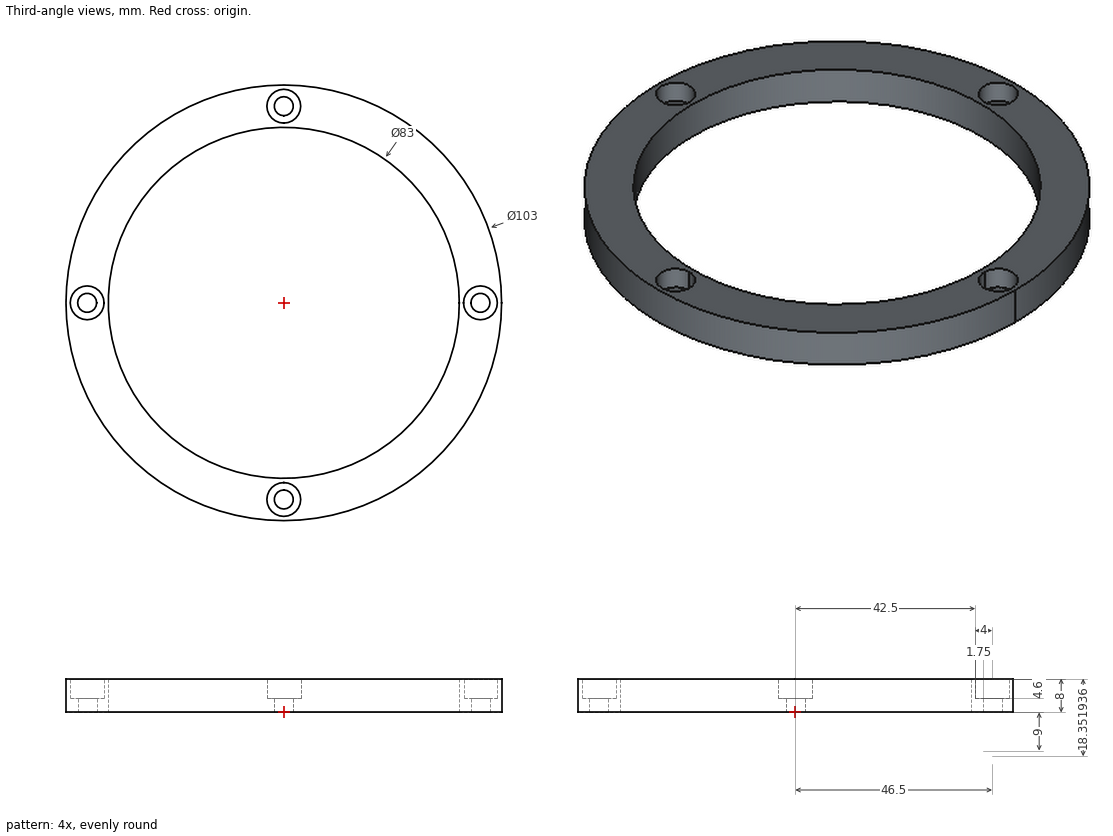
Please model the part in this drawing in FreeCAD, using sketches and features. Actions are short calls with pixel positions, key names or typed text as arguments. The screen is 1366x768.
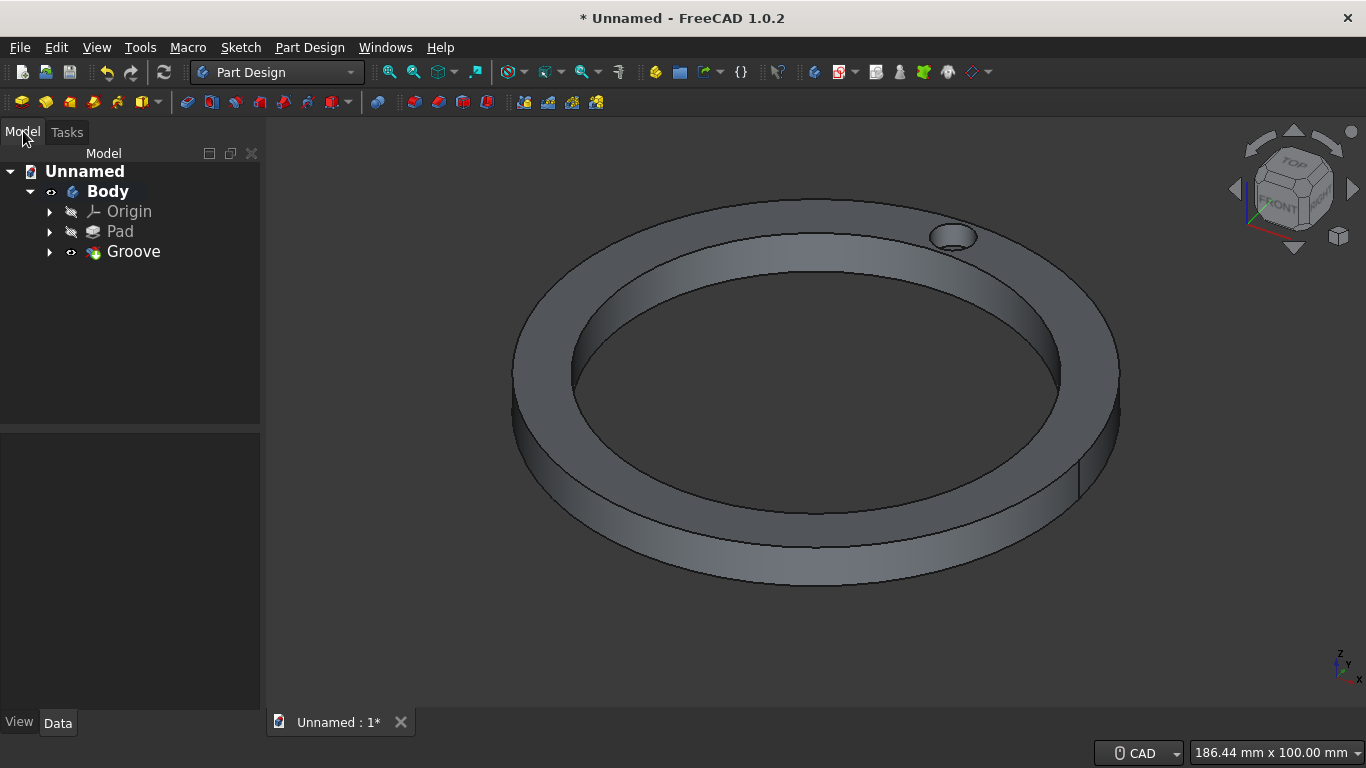
click(116, 252)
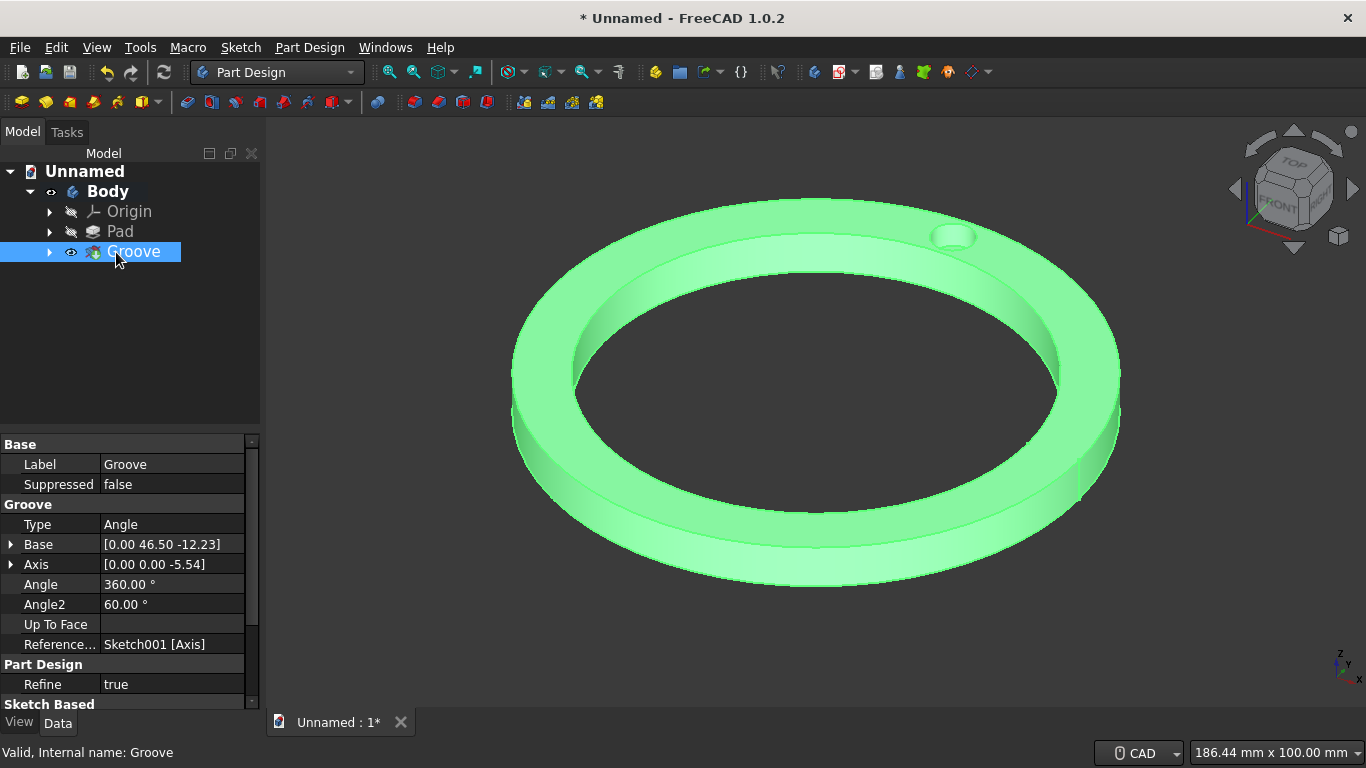
click(572, 102)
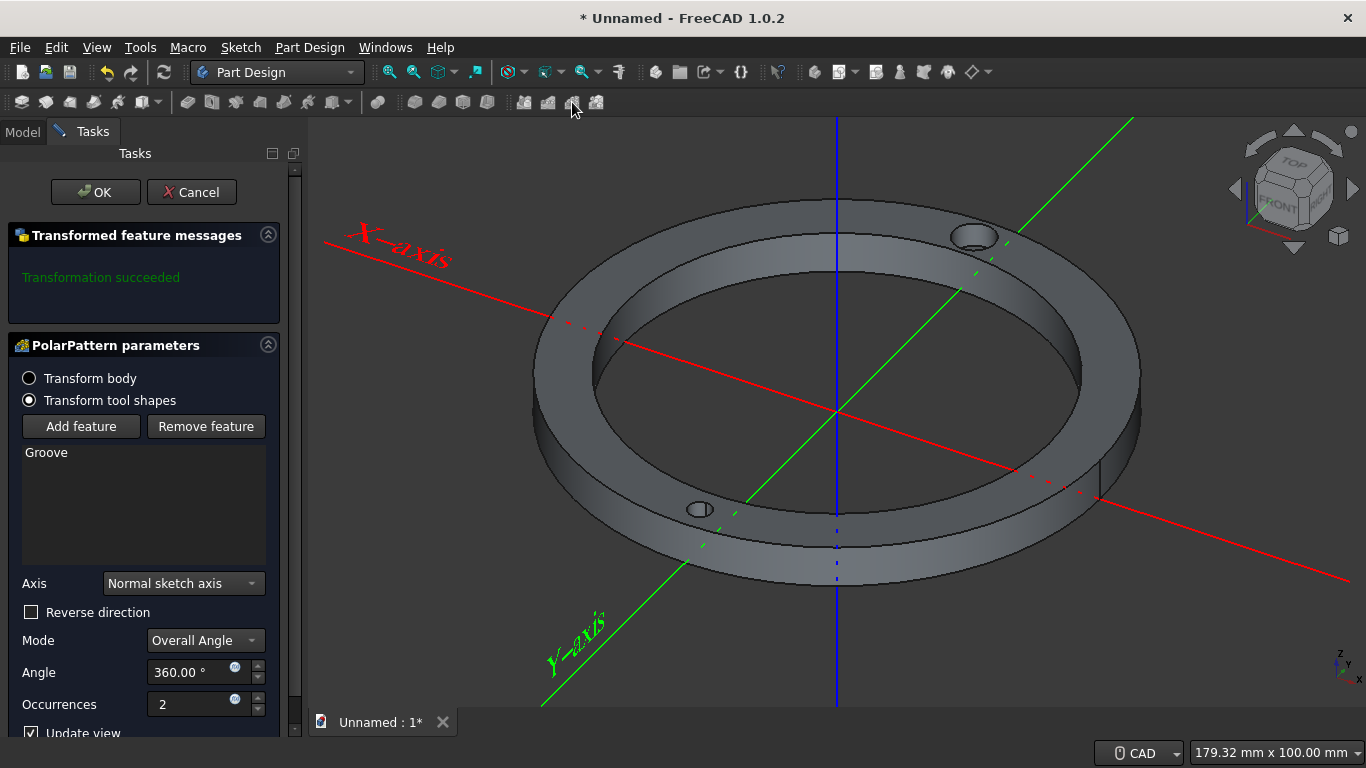
click(184, 584)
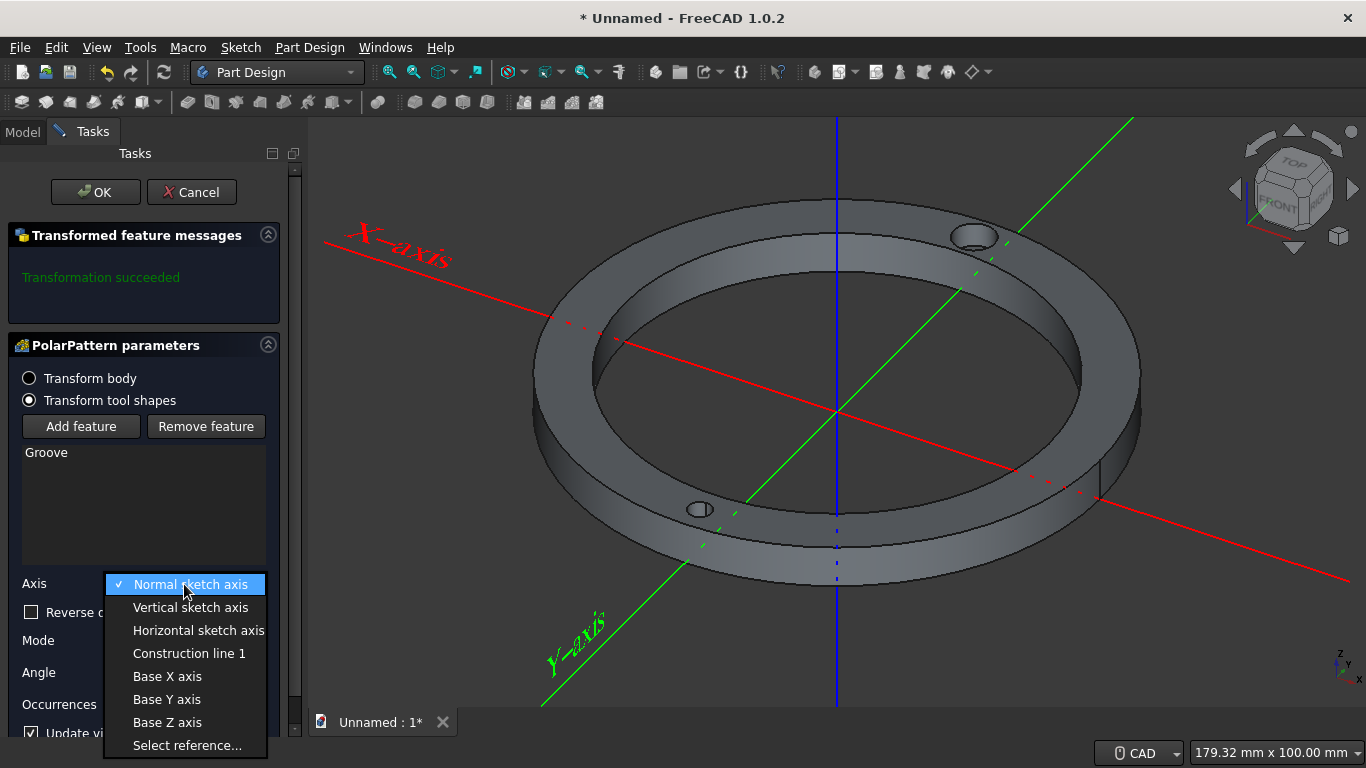
click(184, 722)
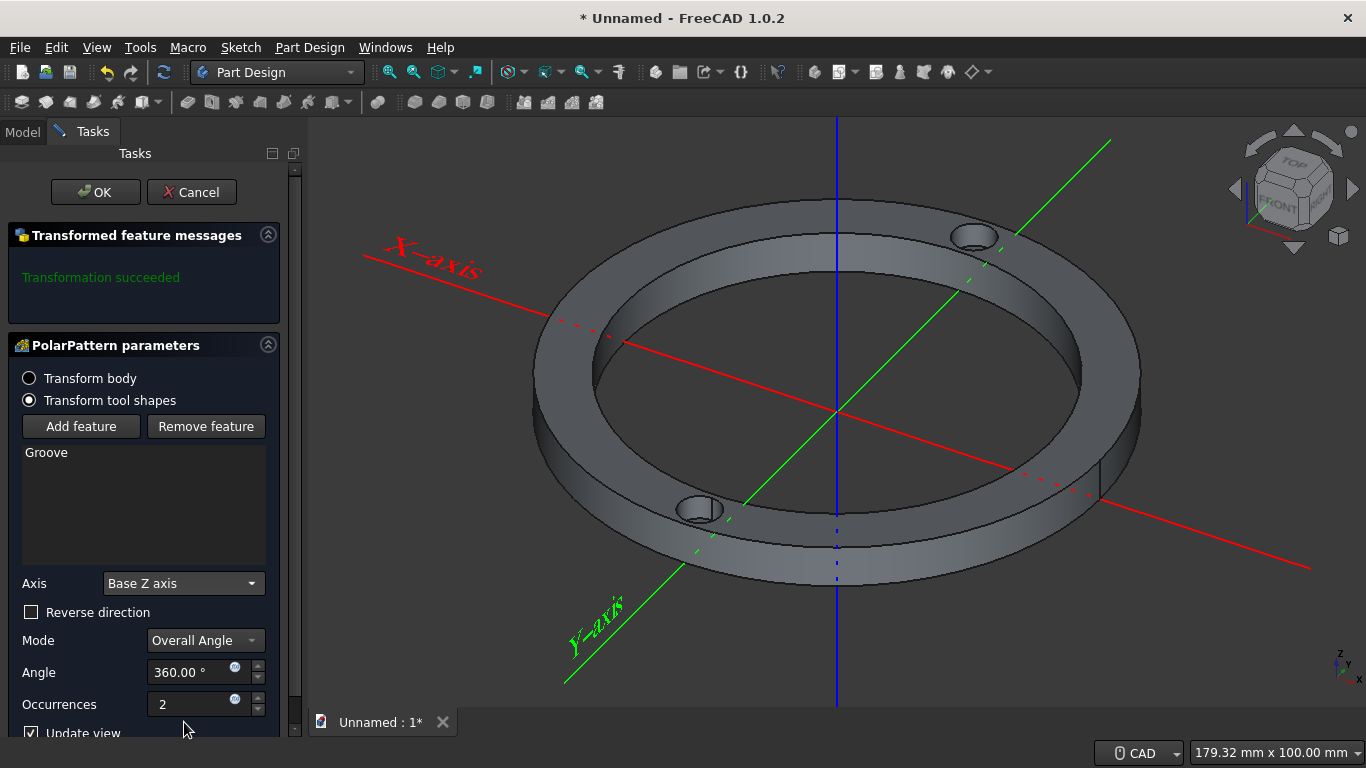
triple_click(198, 704)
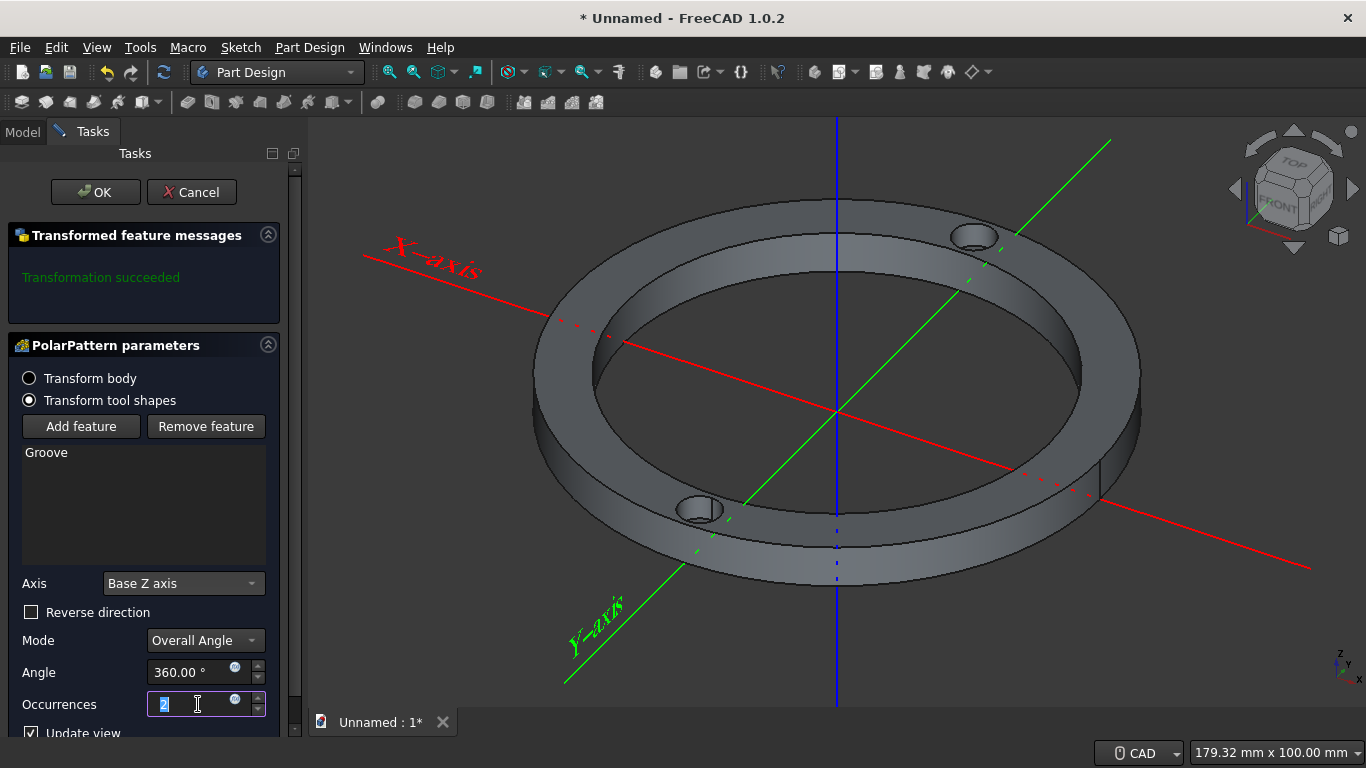
text(4)
key(Tab)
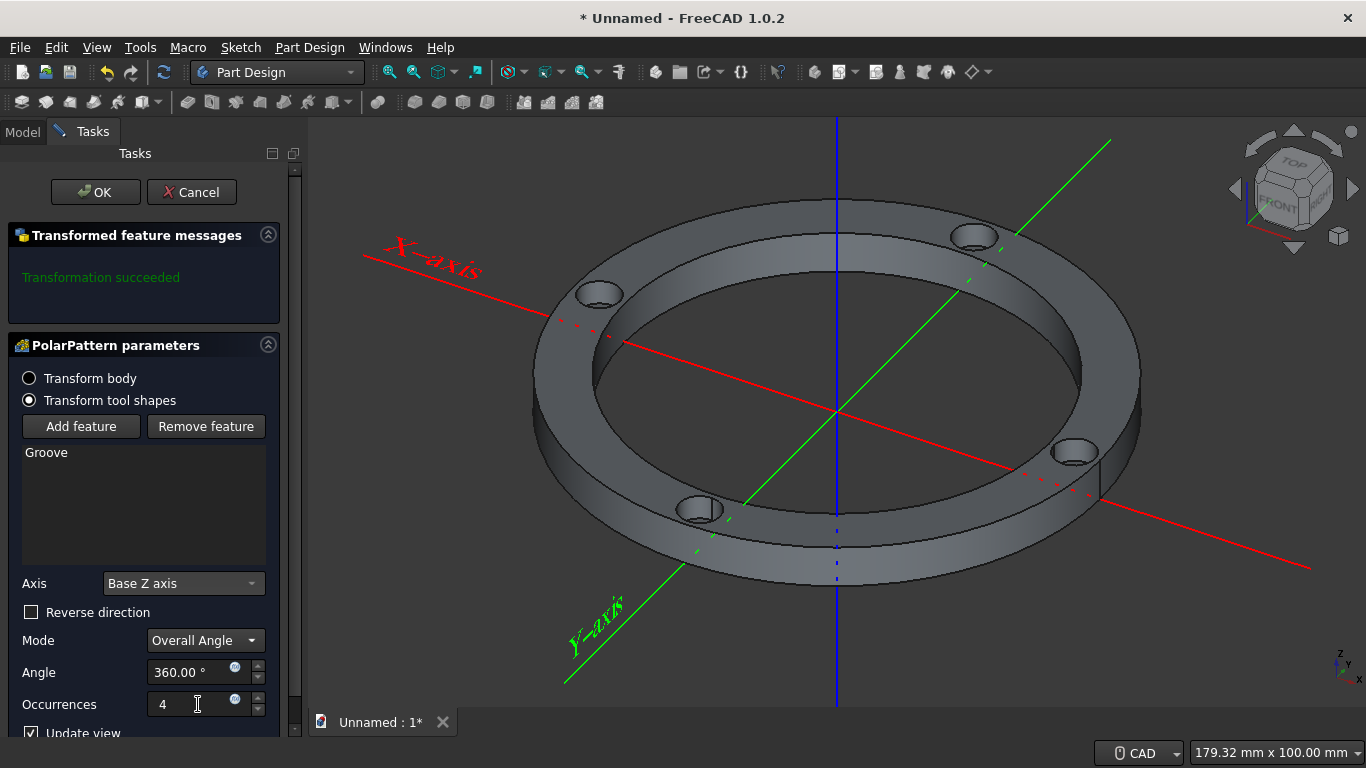
click(96, 192)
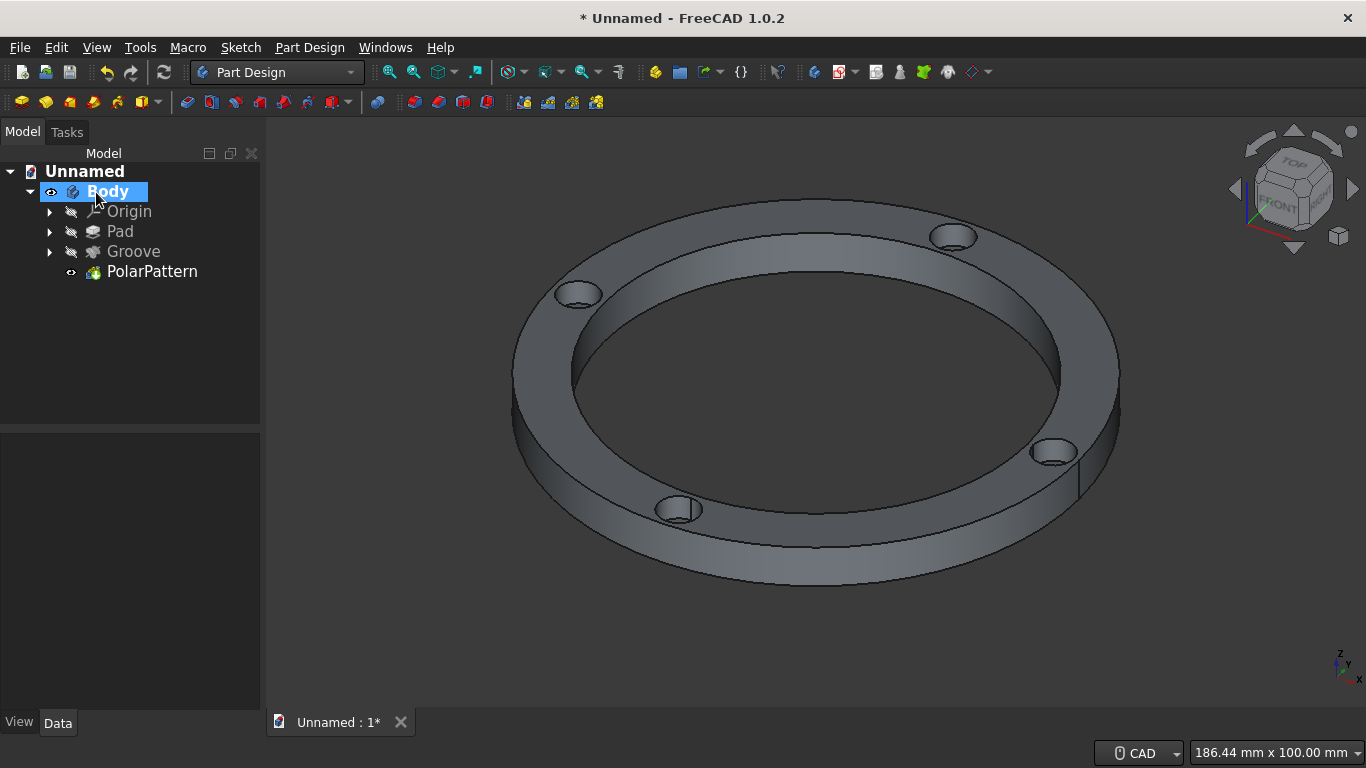
key(0)